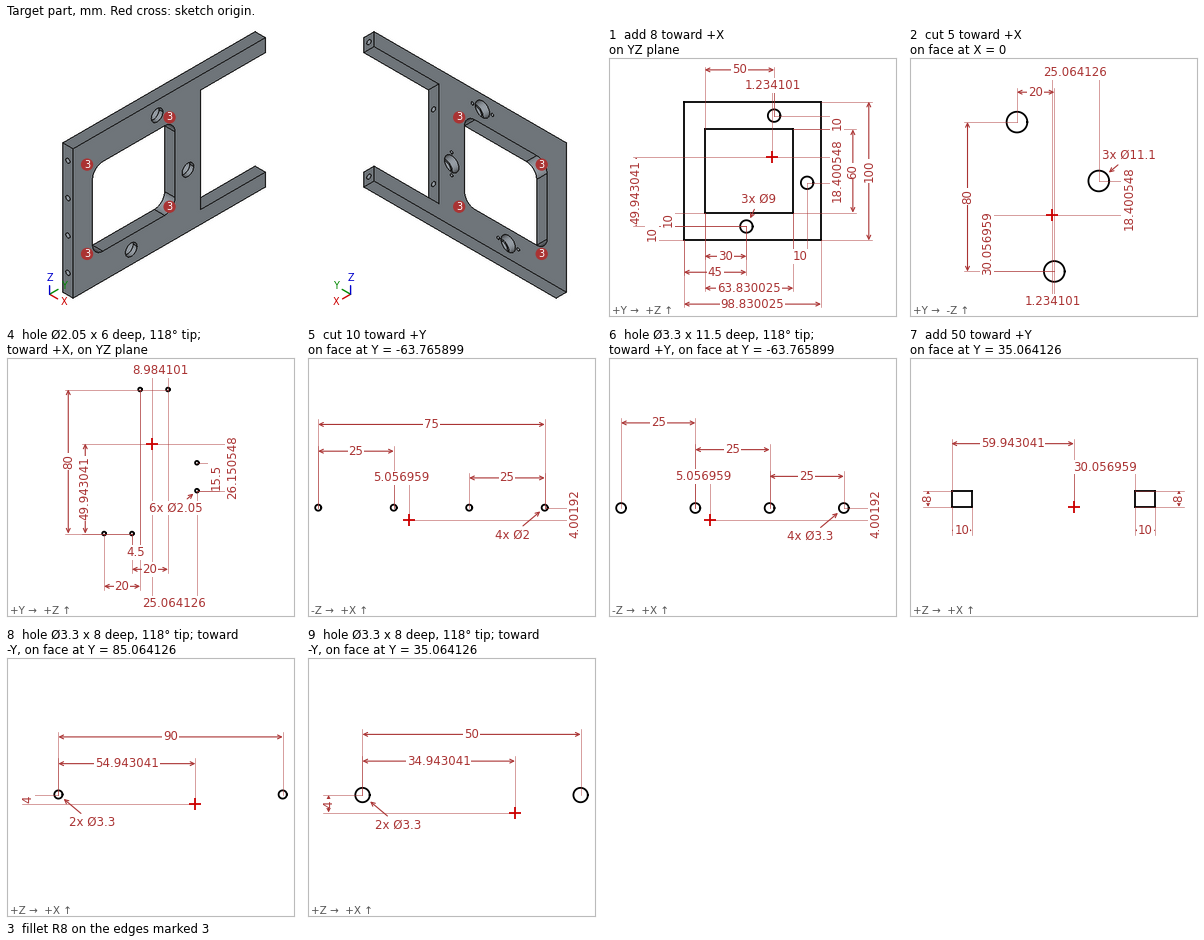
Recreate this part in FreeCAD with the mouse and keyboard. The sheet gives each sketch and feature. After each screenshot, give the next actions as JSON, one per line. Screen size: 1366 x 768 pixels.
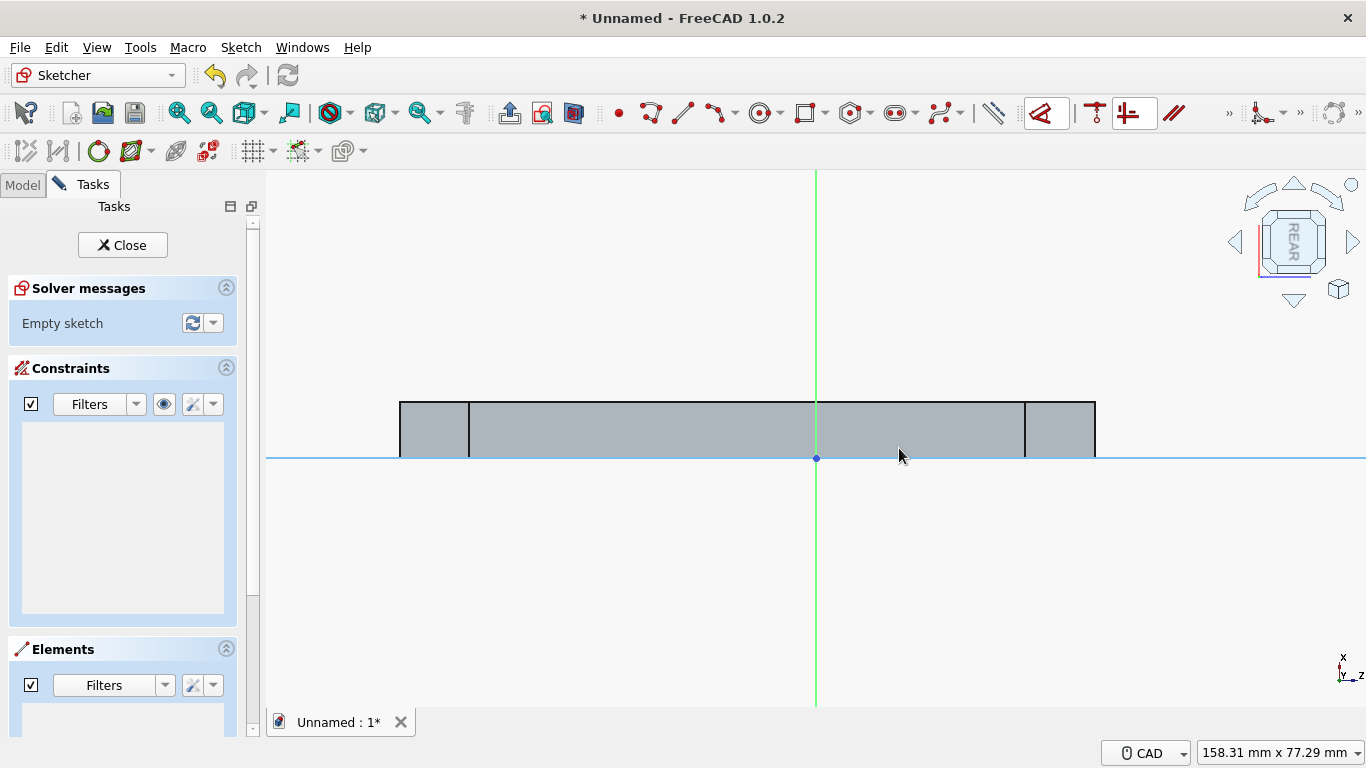
{"action": "left_click", "coordinate": [760, 114]}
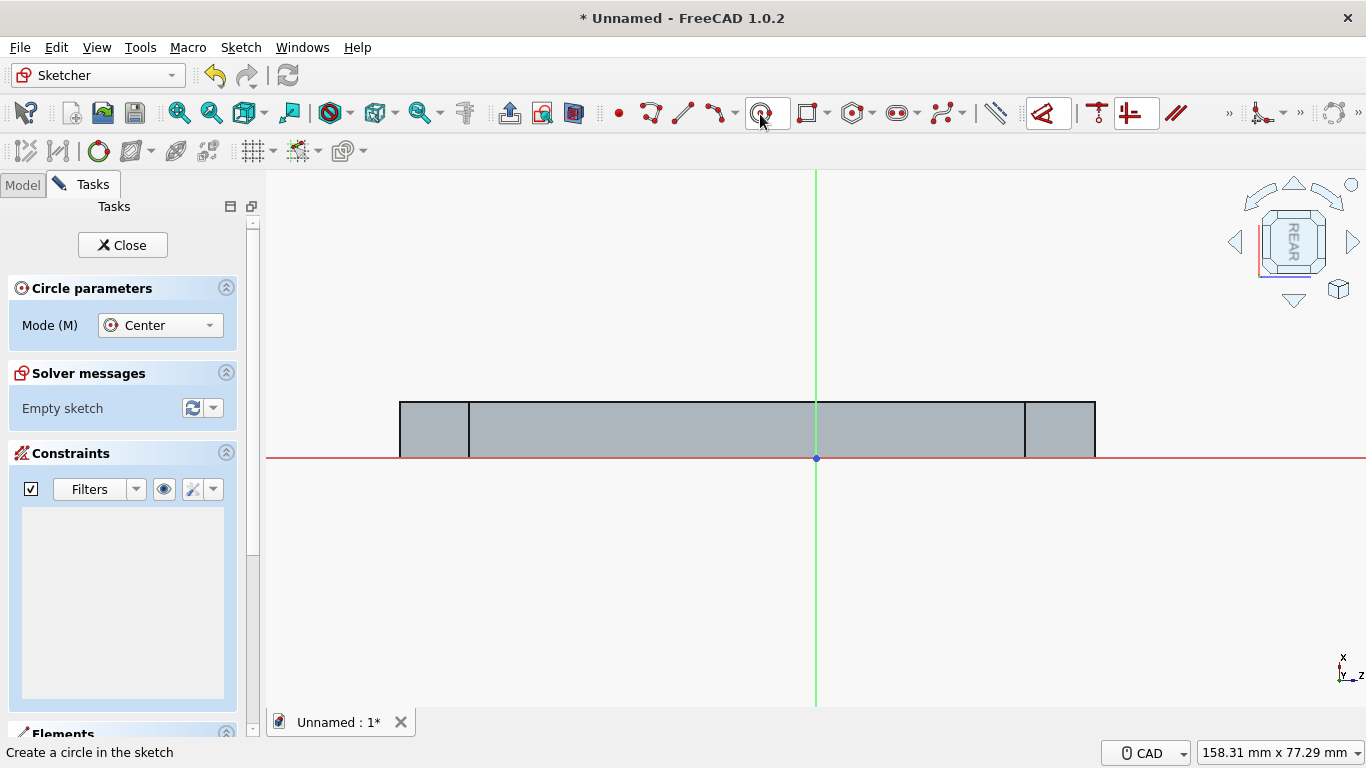
{"action": "scroll", "coordinate": [435, 430], "scroll_direction": "up", "scroll_amount": 4}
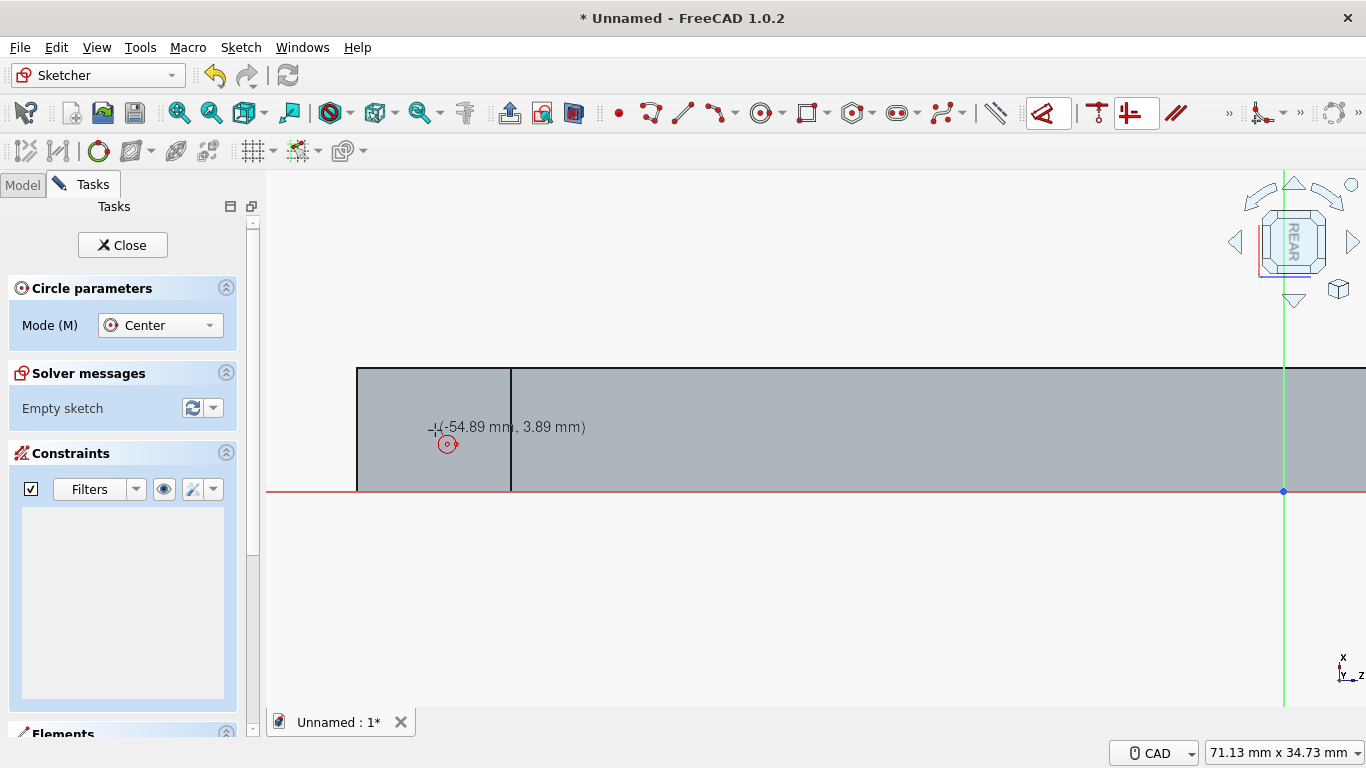
{"action": "left_click", "coordinate": [434, 430]}
{"action": "mouse_move", "coordinate": [452, 412]}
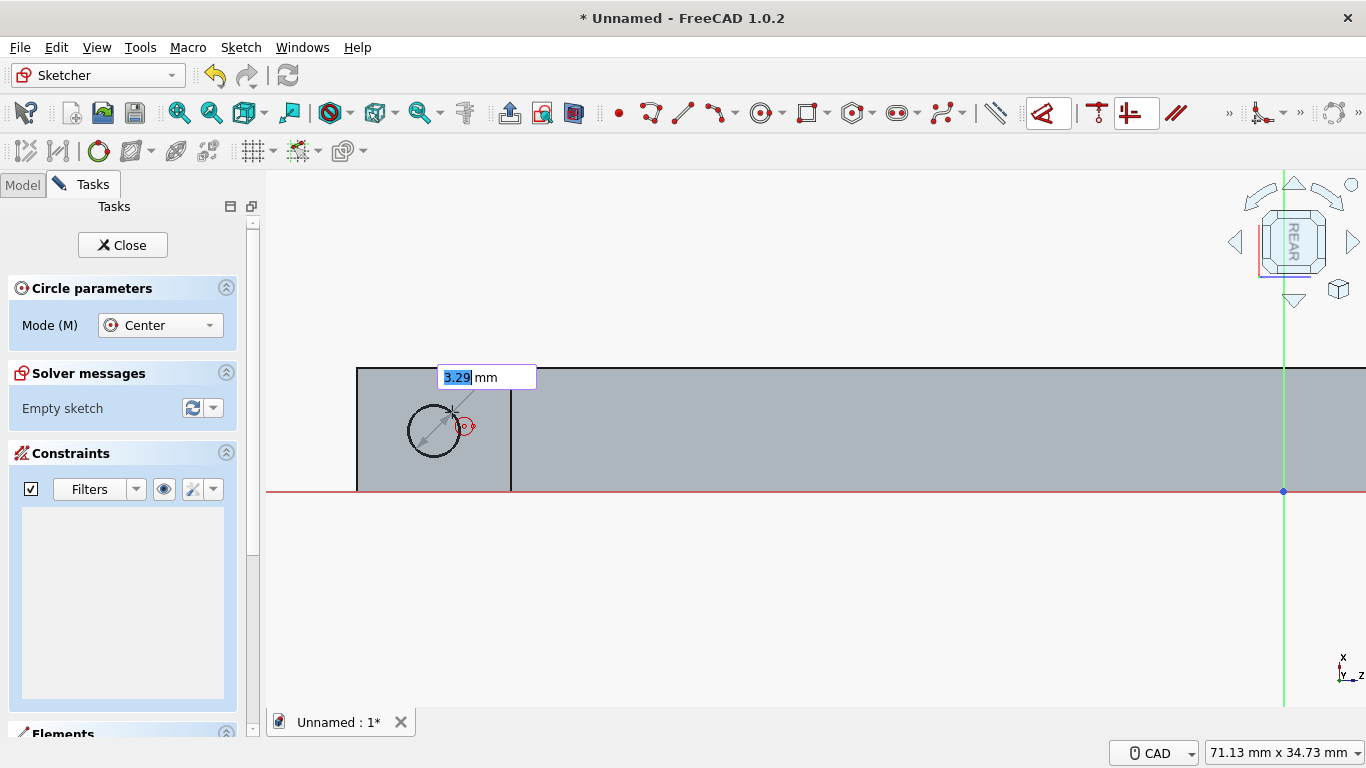
{"action": "type", "text": "3.3"}
{"action": "key", "text": "Return"}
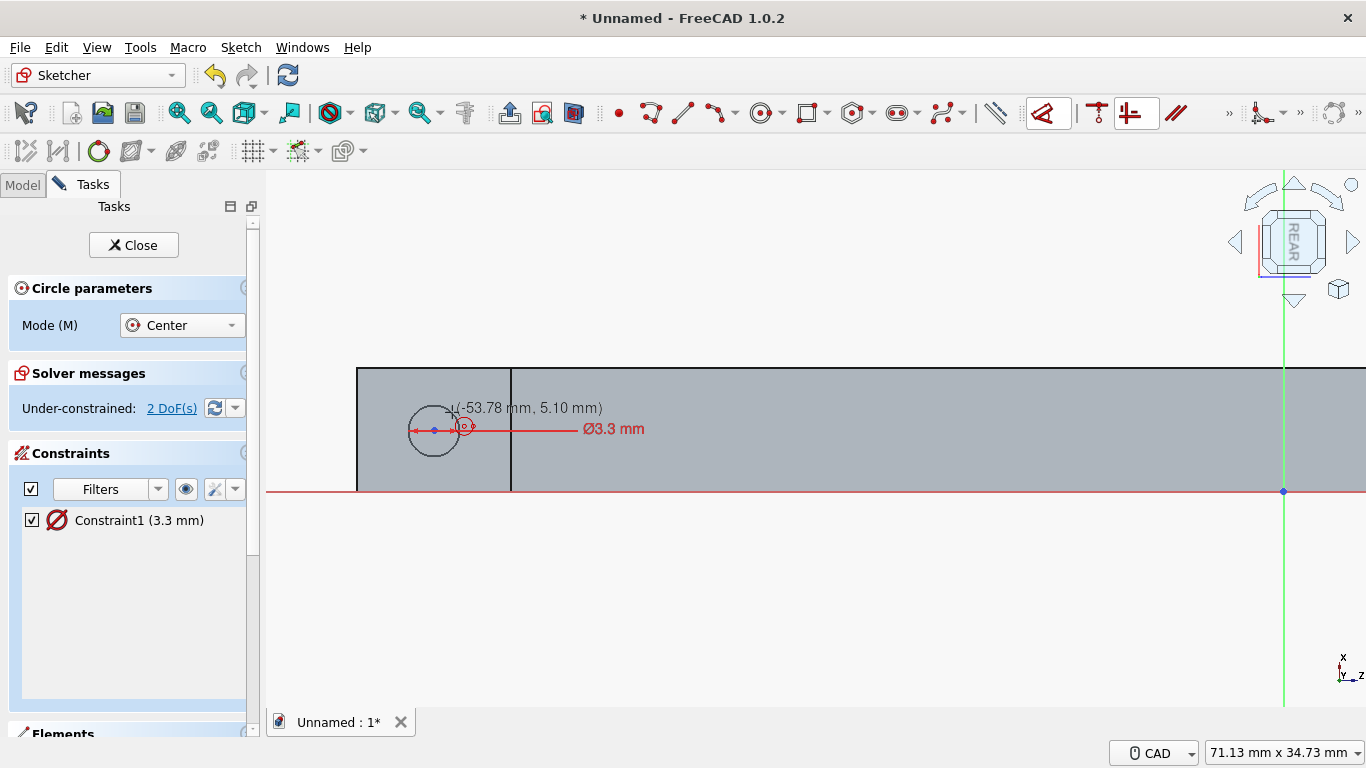
{"action": "scroll", "coordinate": [436, 431], "scroll_direction": "down", "scroll_amount": 4}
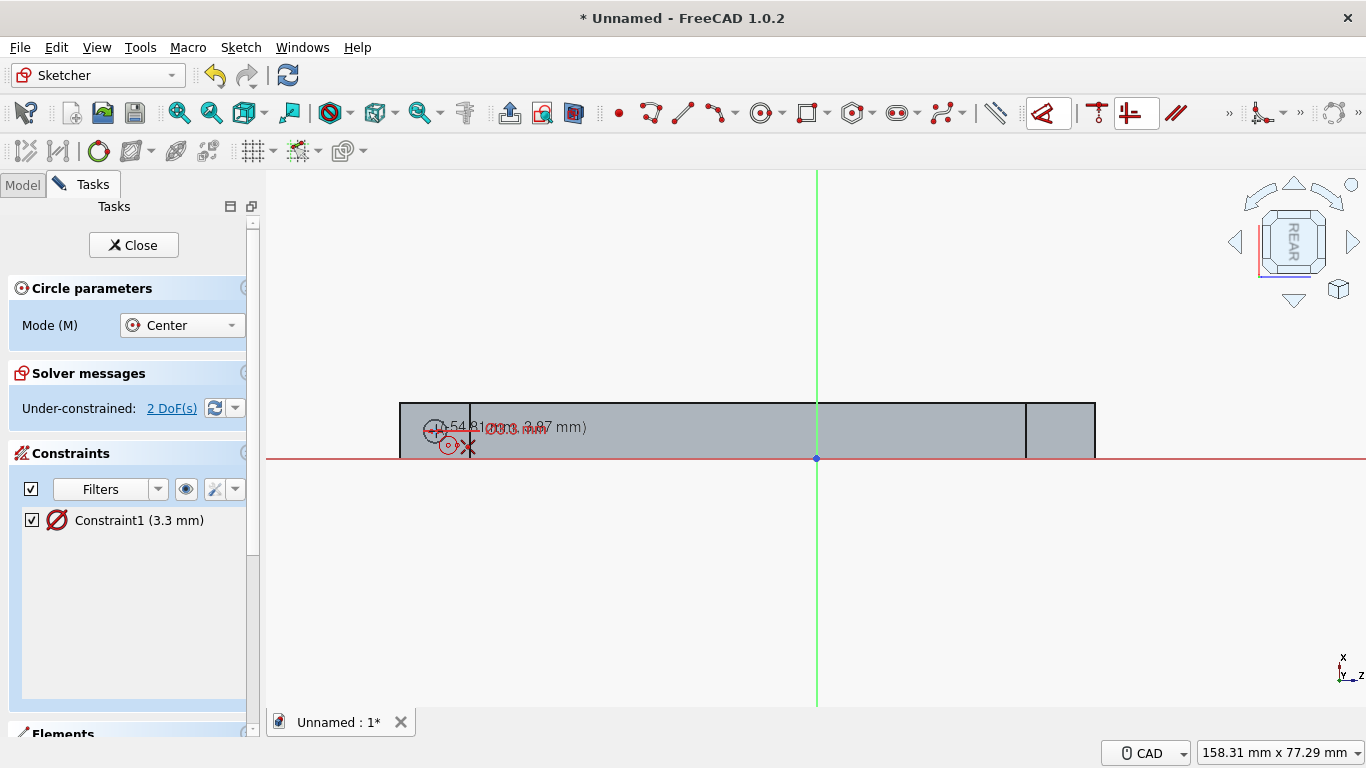
{"action": "scroll", "coordinate": [1061, 431], "scroll_direction": "up", "scroll_amount": 4}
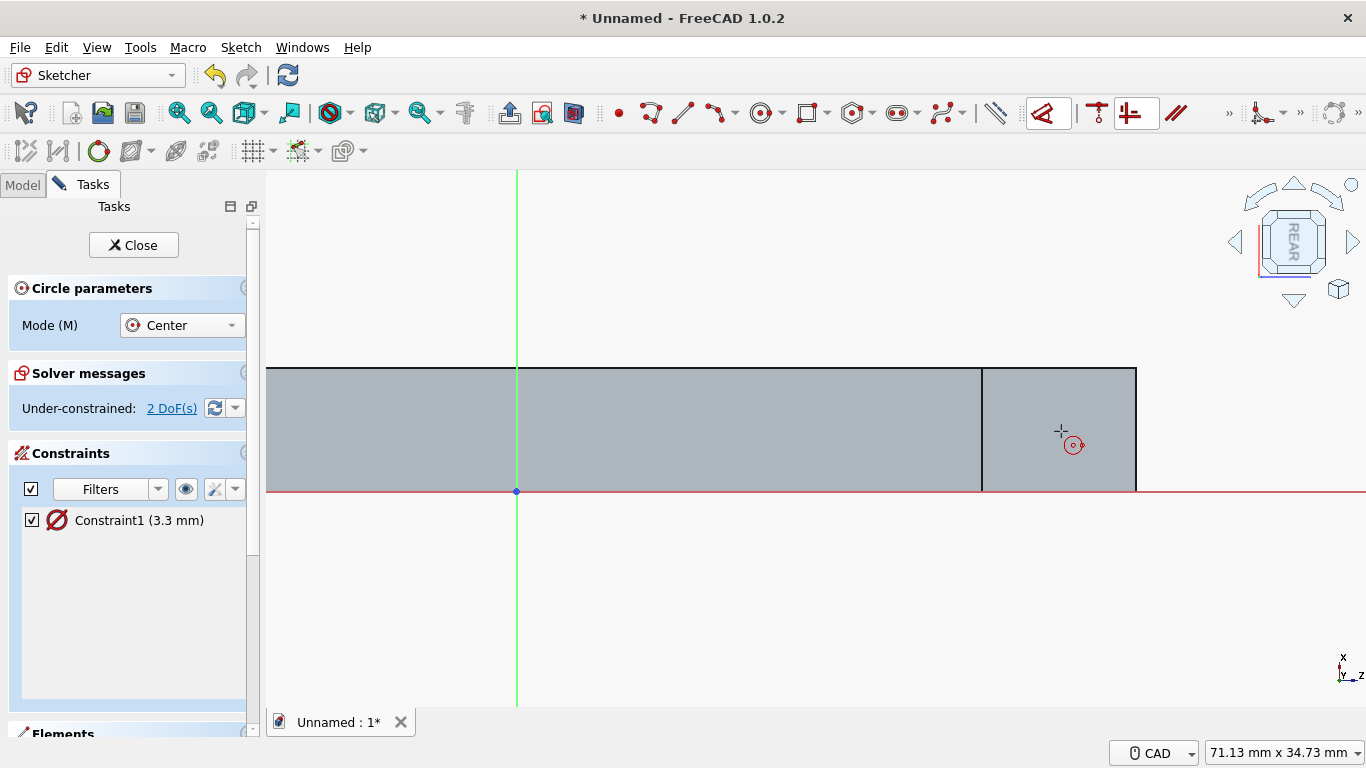
{"action": "left_click", "coordinate": [1059, 430]}
{"action": "mouse_move", "coordinate": [1077, 412]}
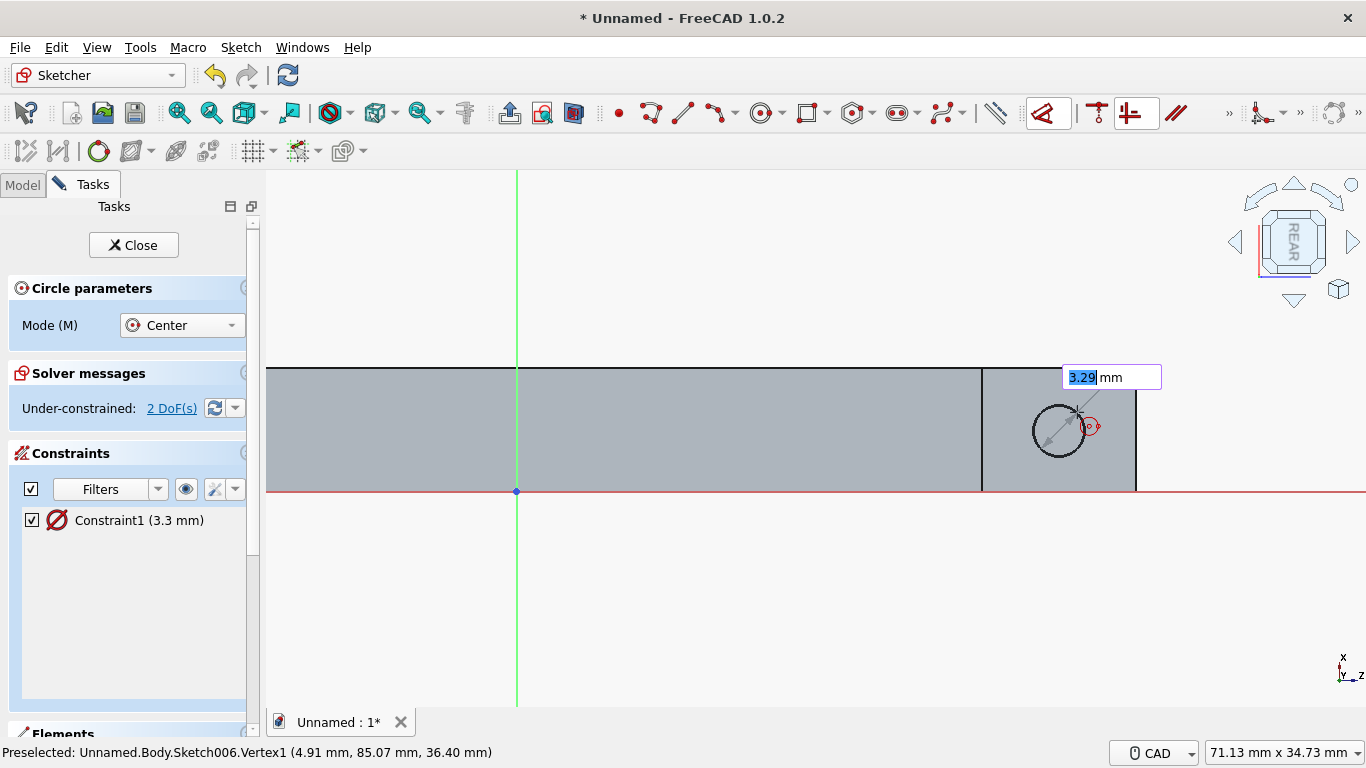
{"action": "type", "text": "3.3"}
{"action": "key", "text": "Return"}
{"action": "key", "text": "Escape"}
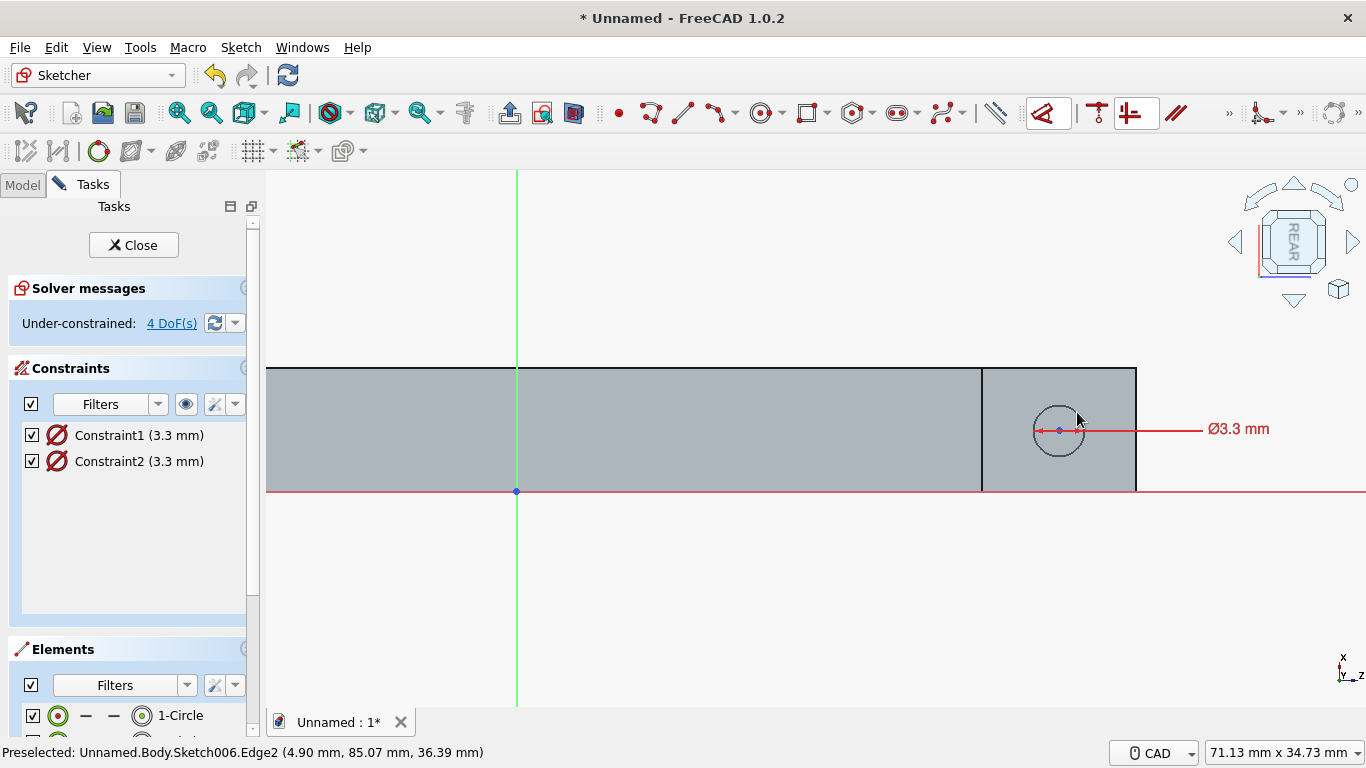
{"action": "scroll", "coordinate": [1061, 431], "scroll_direction": "down", "scroll_amount": 4}